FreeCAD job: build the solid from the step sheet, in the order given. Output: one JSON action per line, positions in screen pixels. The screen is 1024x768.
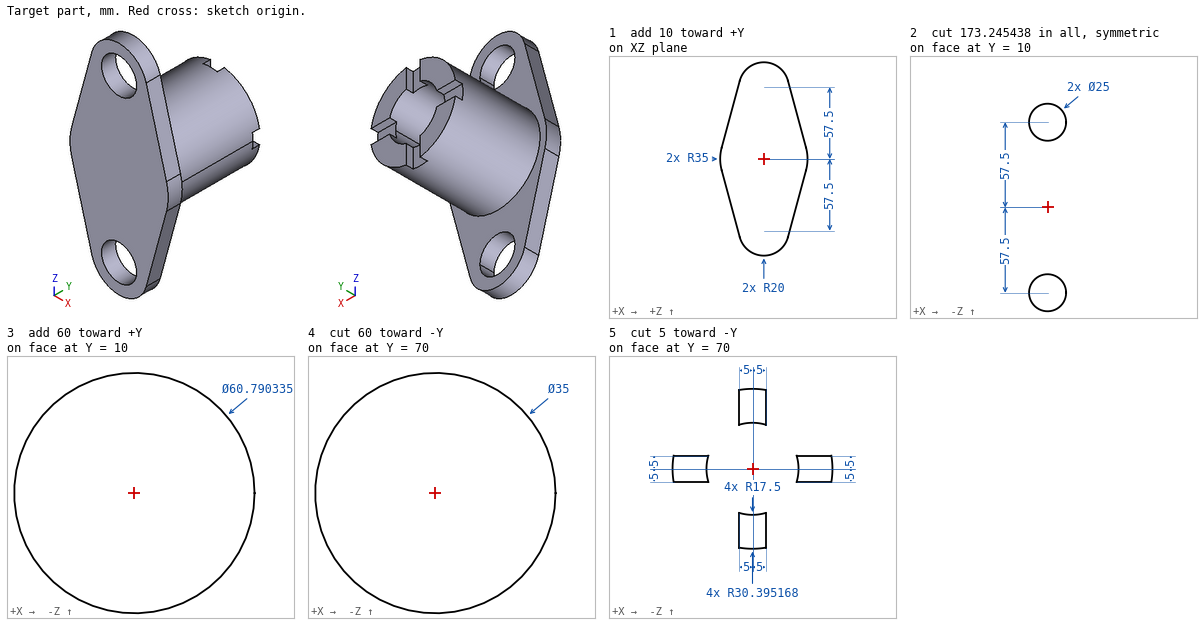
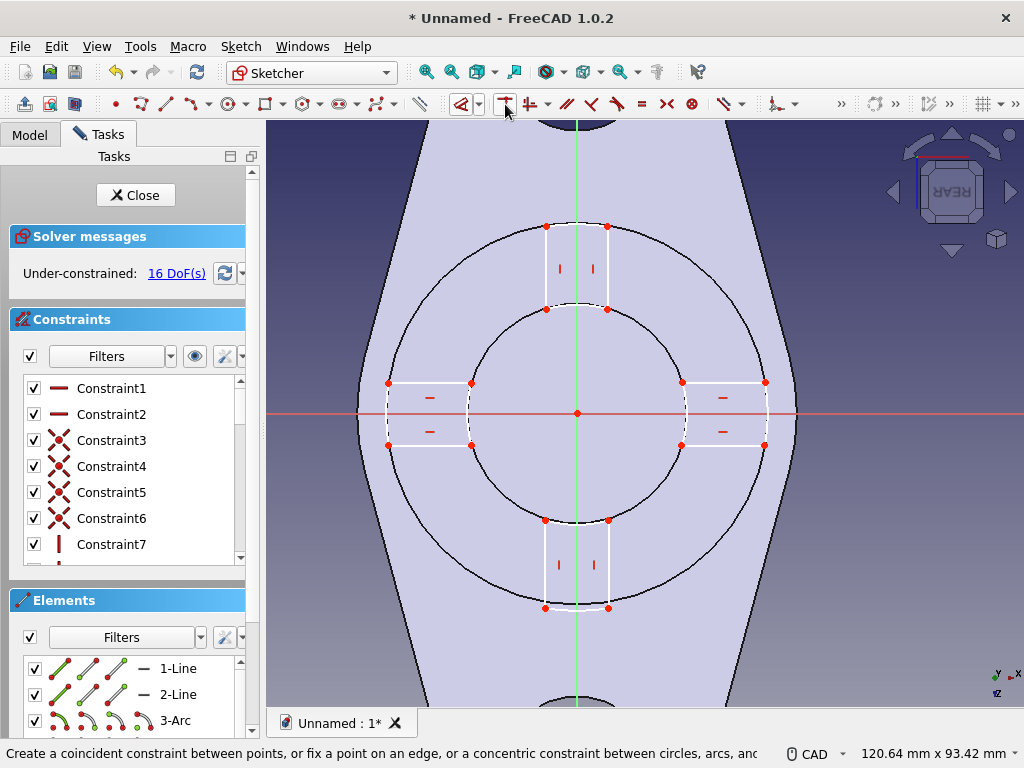
{"action": "left_click", "coordinate": [387, 402]}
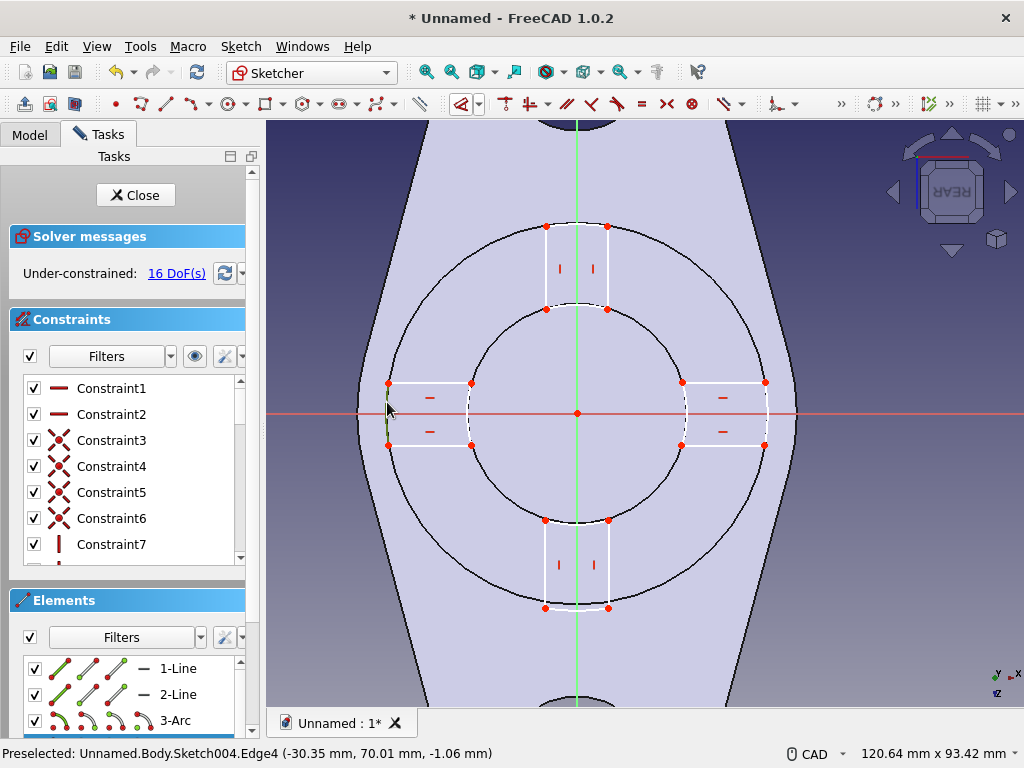
{"action": "left_click", "coordinate": [564, 610]}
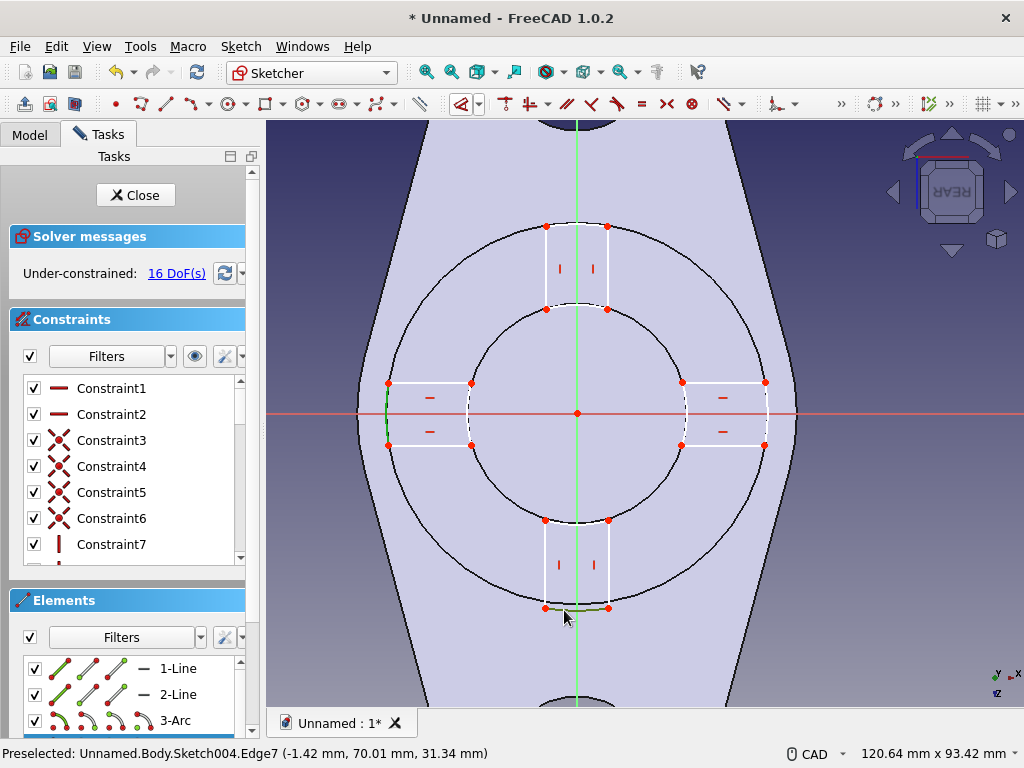
{"action": "left_click", "coordinate": [589, 225]}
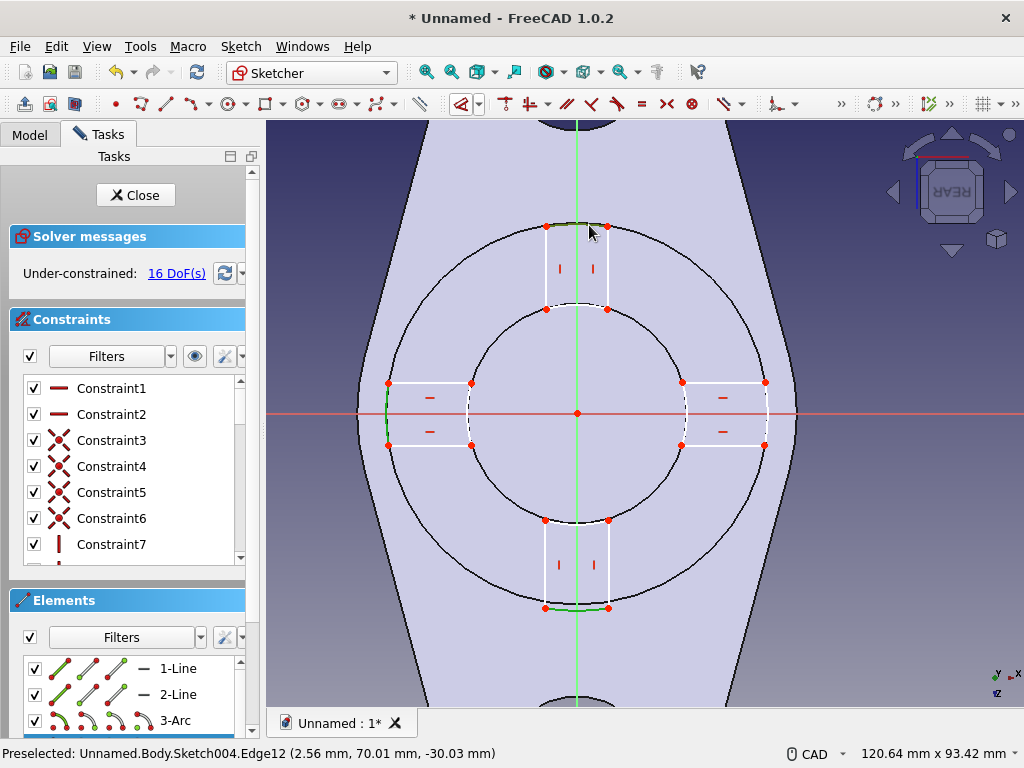
{"action": "left_click", "coordinate": [767, 427]}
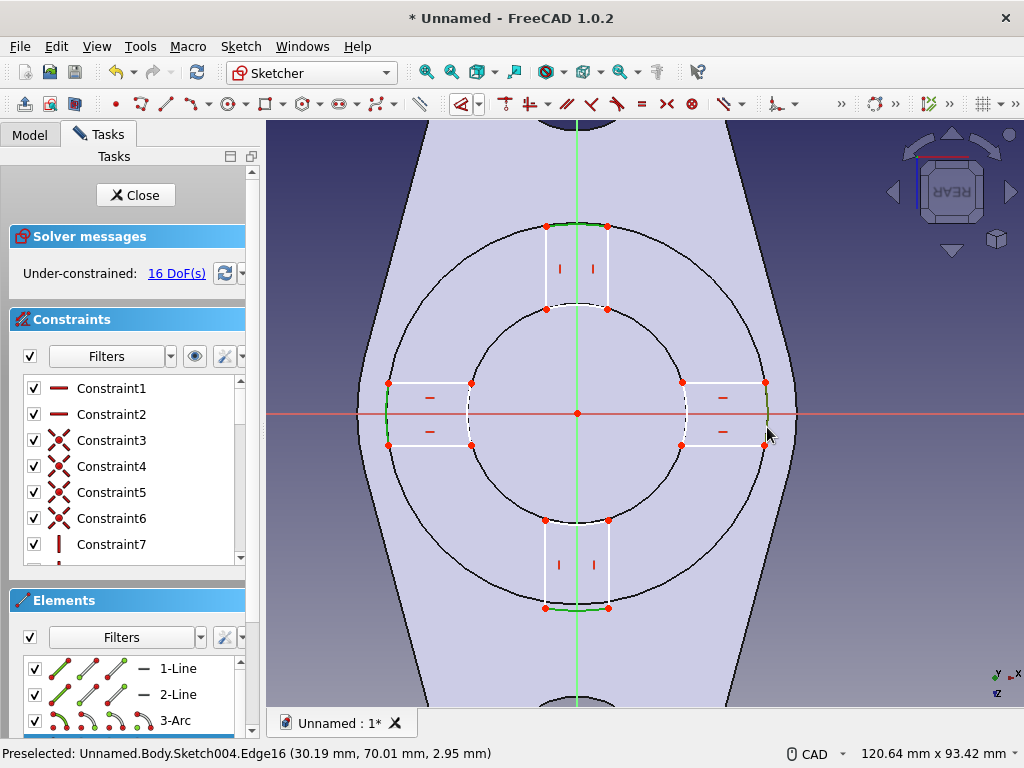
{"action": "left_click", "coordinate": [642, 104]}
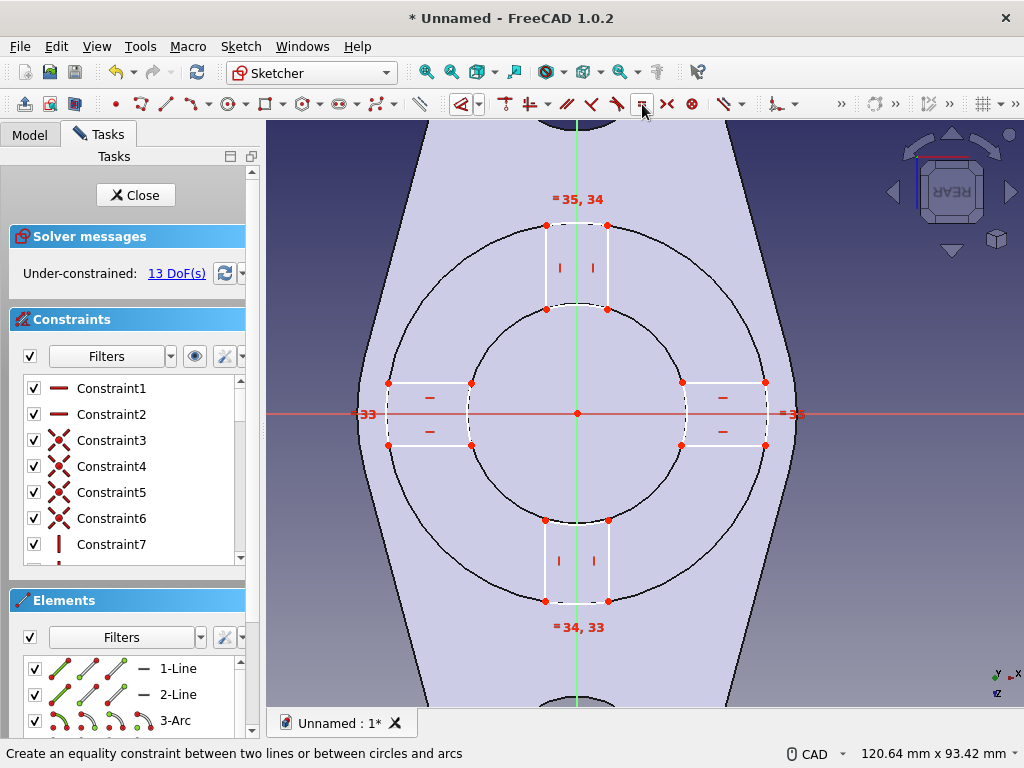
{"action": "left_click", "coordinate": [468, 402]}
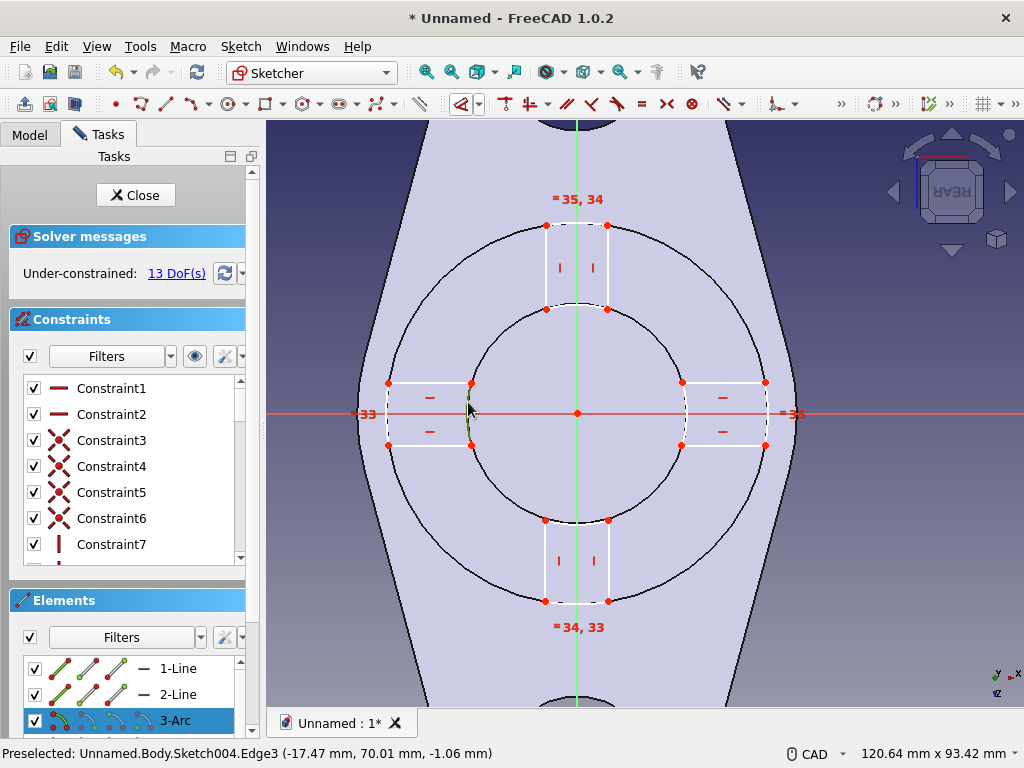
{"action": "left_click", "coordinate": [564, 524]}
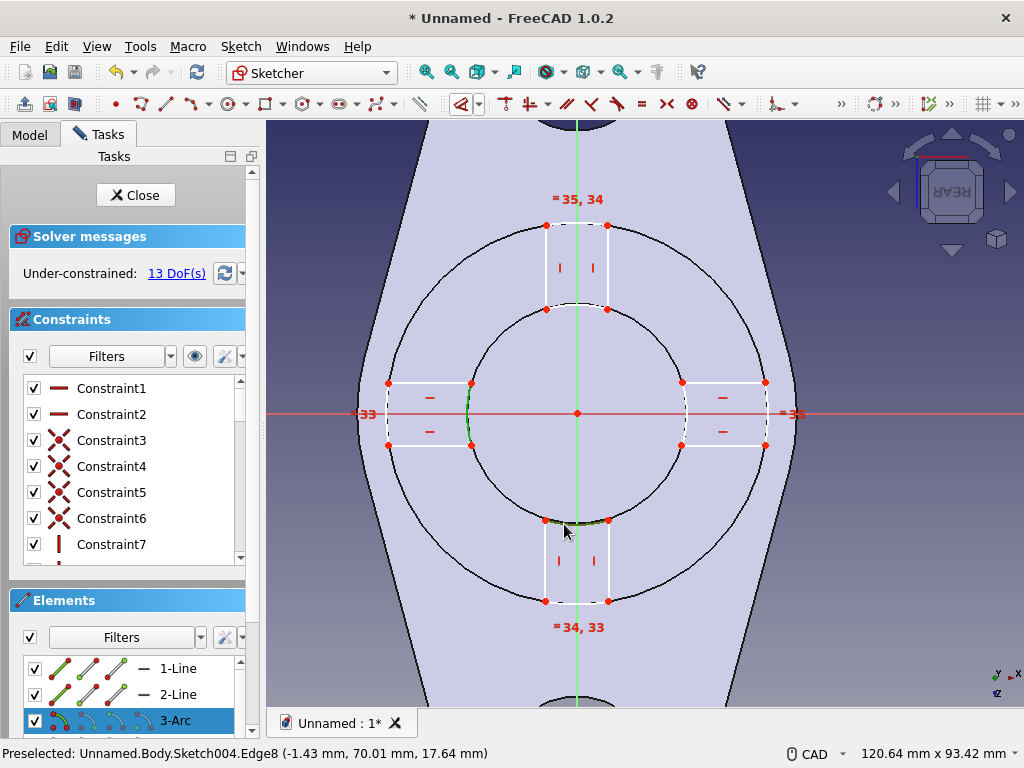
{"action": "left_click", "coordinate": [590, 306]}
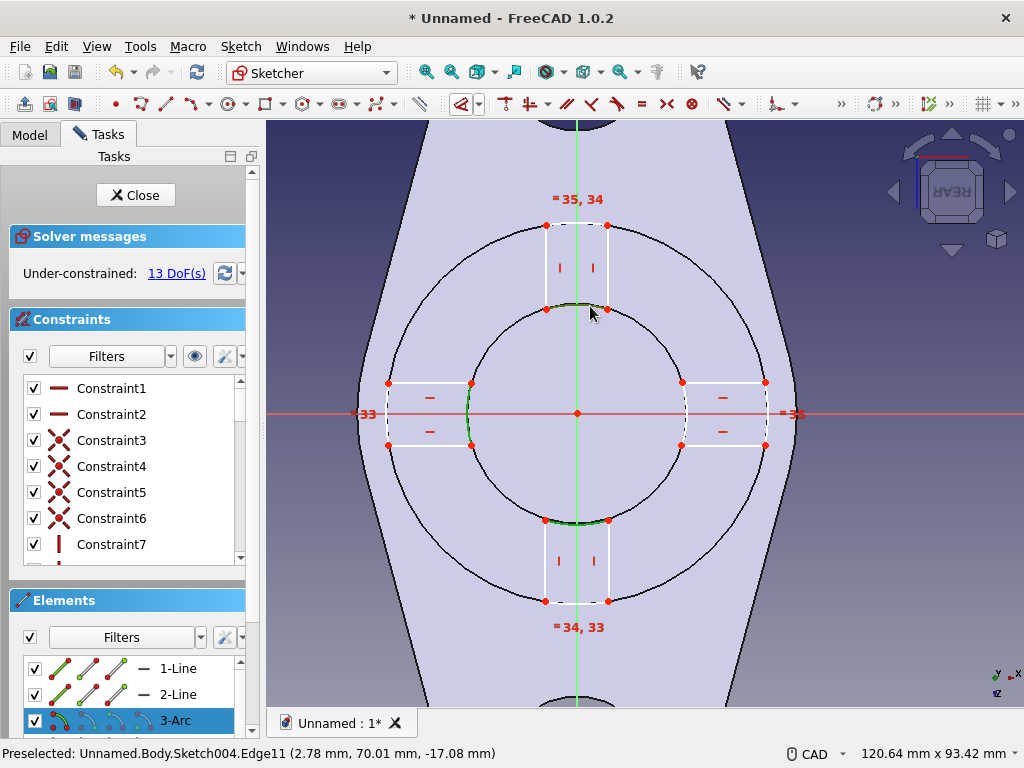
{"action": "left_click", "coordinate": [686, 427]}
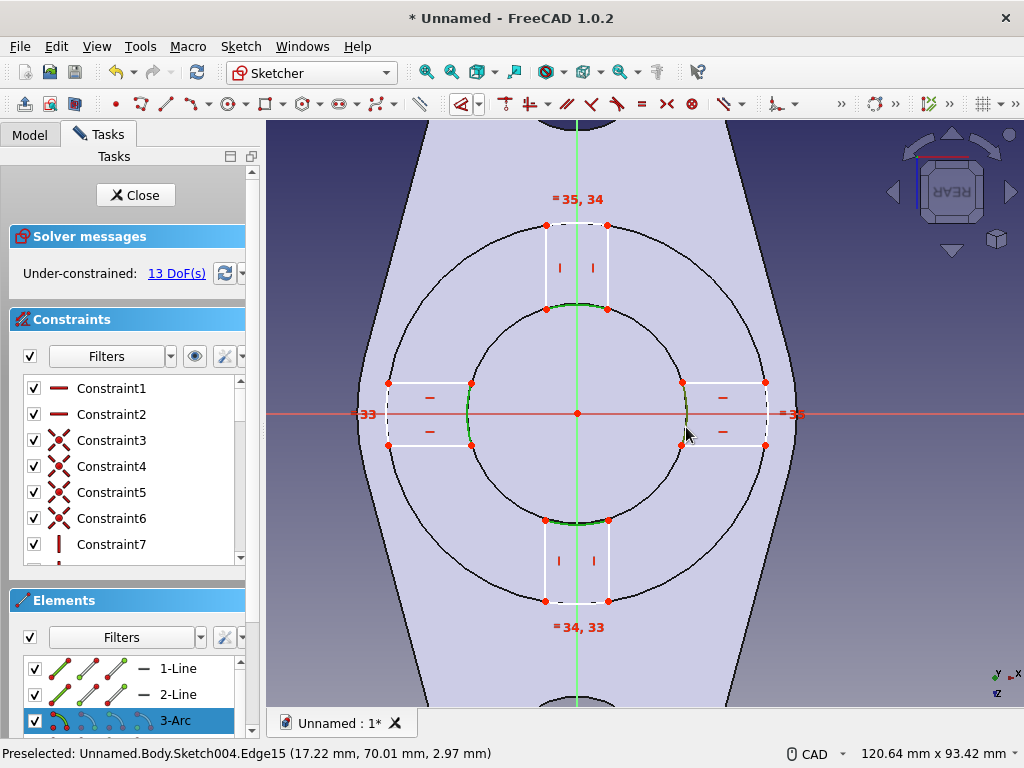
{"action": "left_click", "coordinate": [642, 104]}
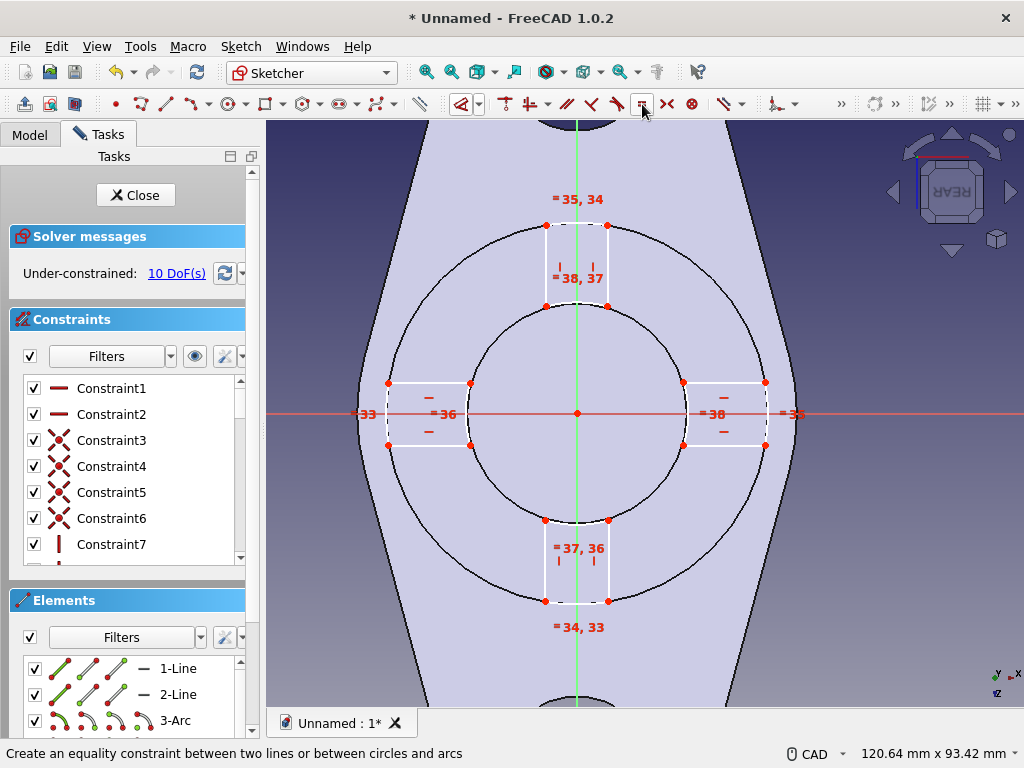
{"action": "left_click", "coordinate": [466, 402]}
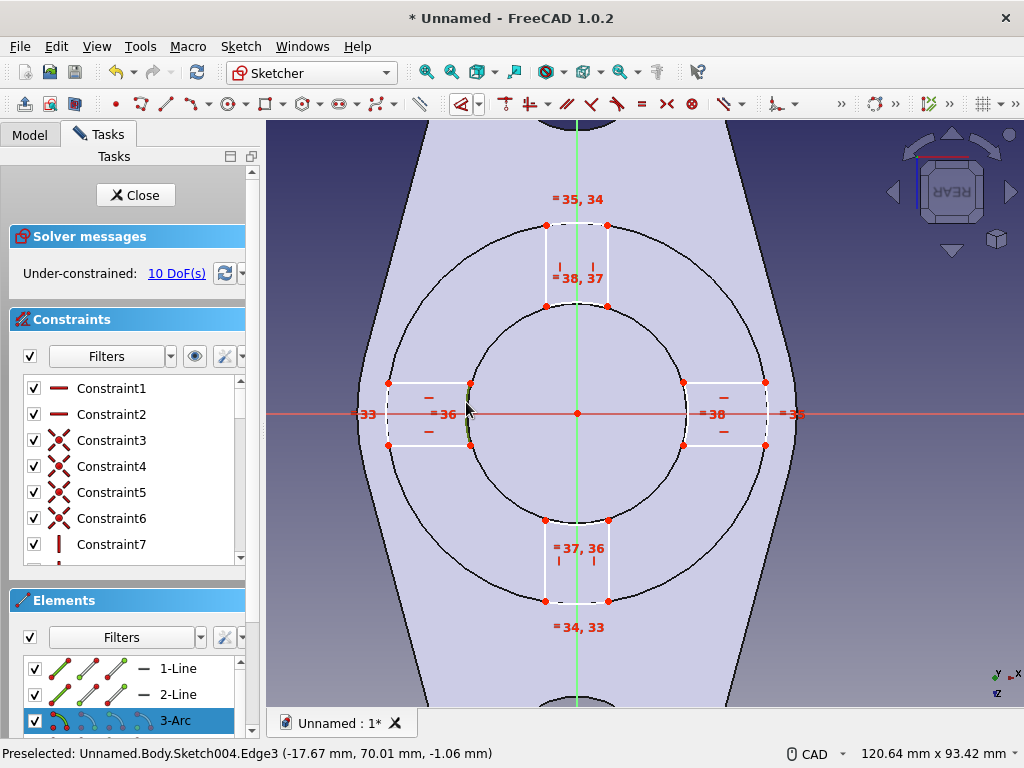
{"action": "key", "text": "k r"}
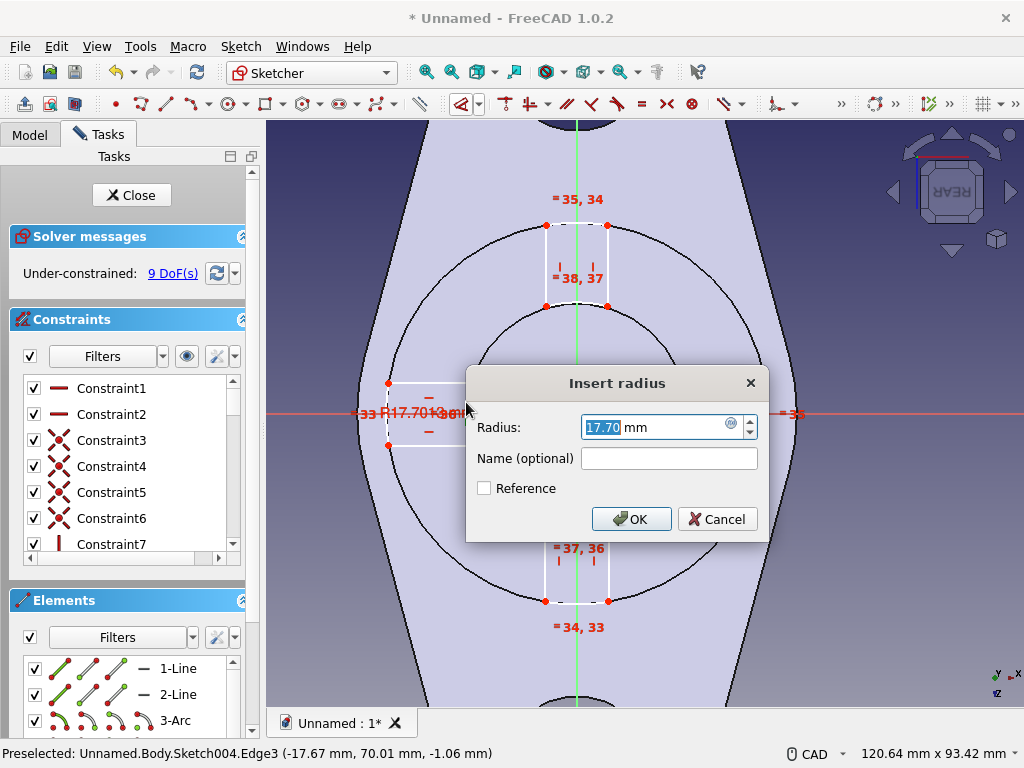
{"action": "type", "text": "17.5"}
{"action": "key", "text": "Return"}